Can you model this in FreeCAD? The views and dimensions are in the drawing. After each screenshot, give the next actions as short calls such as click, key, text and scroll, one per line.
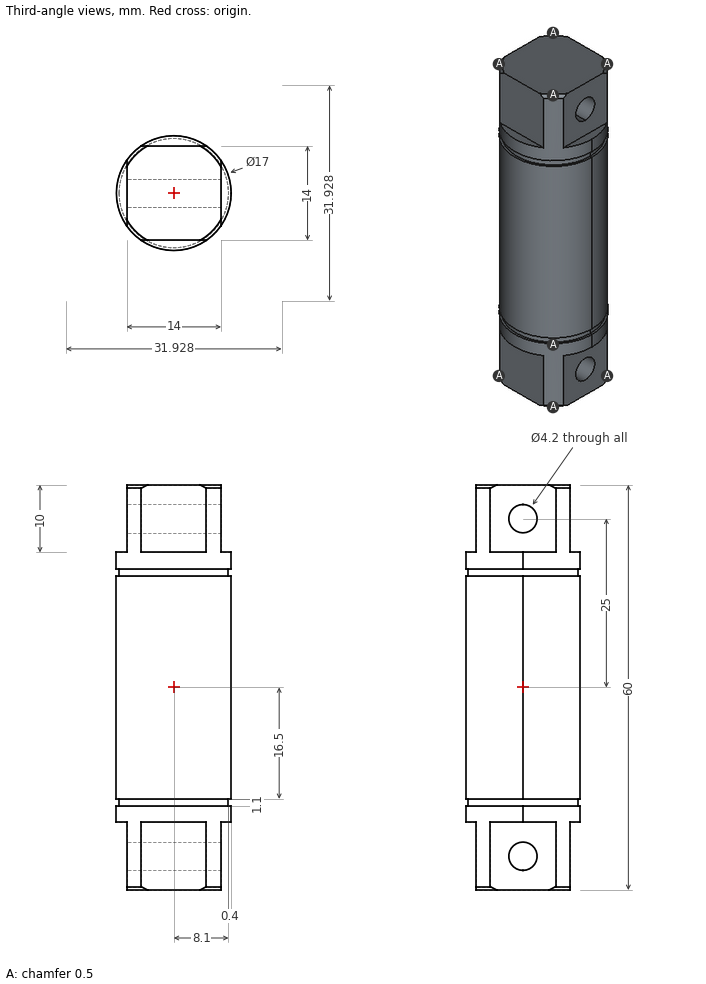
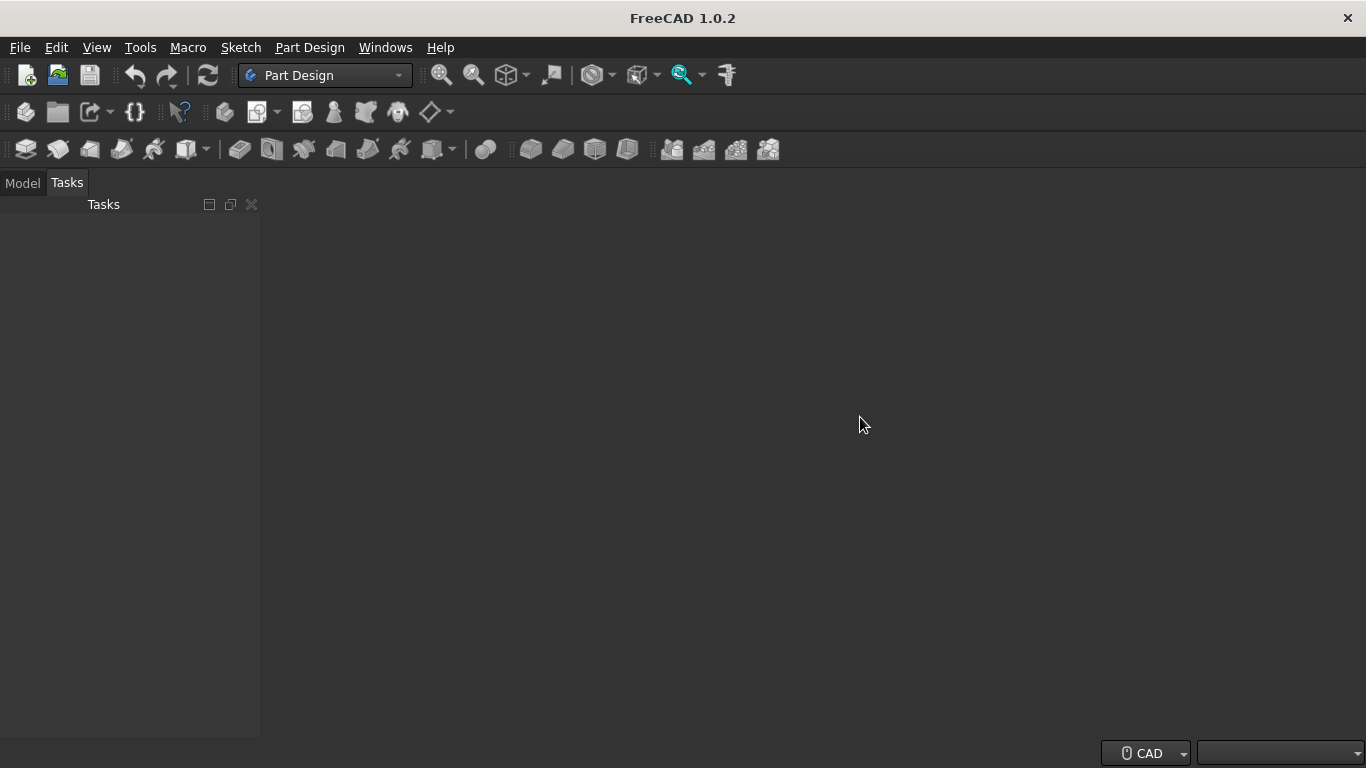
key(ctrl+n)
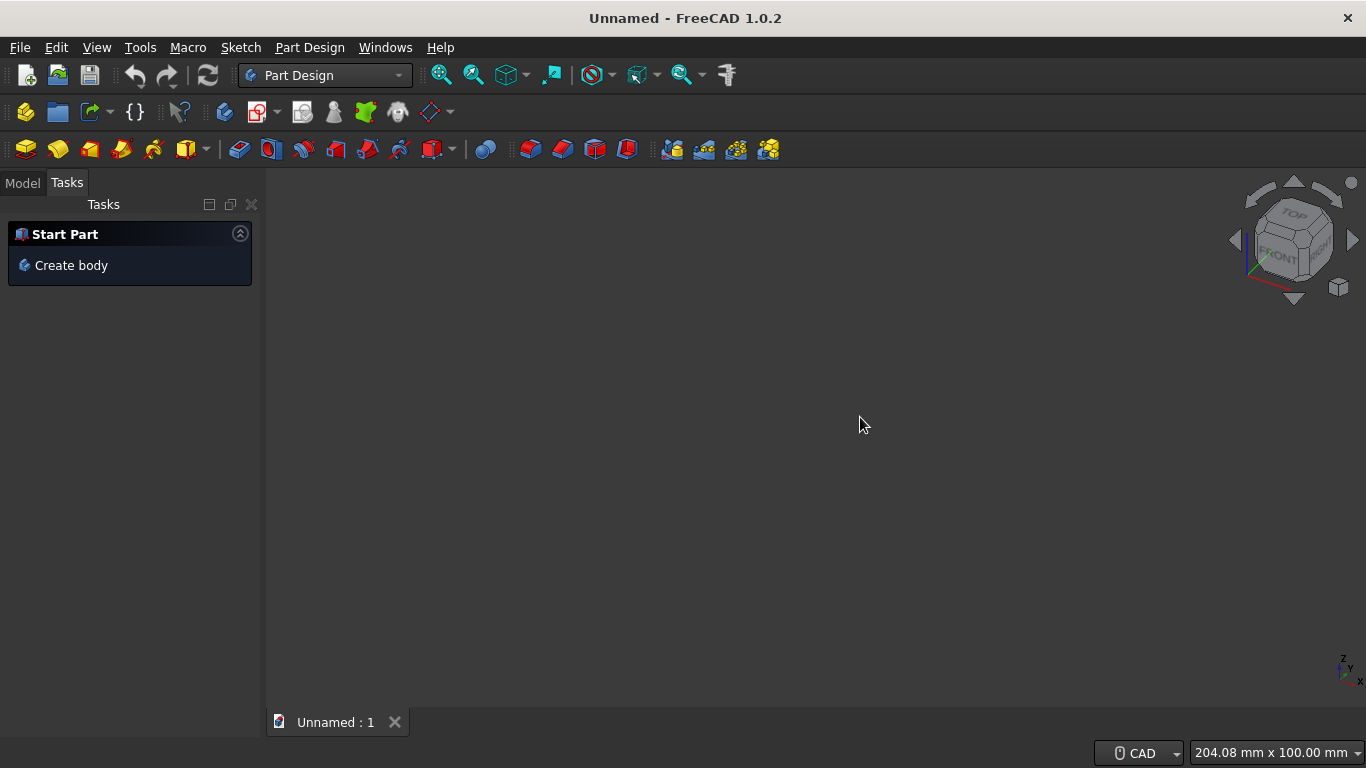
click(258, 112)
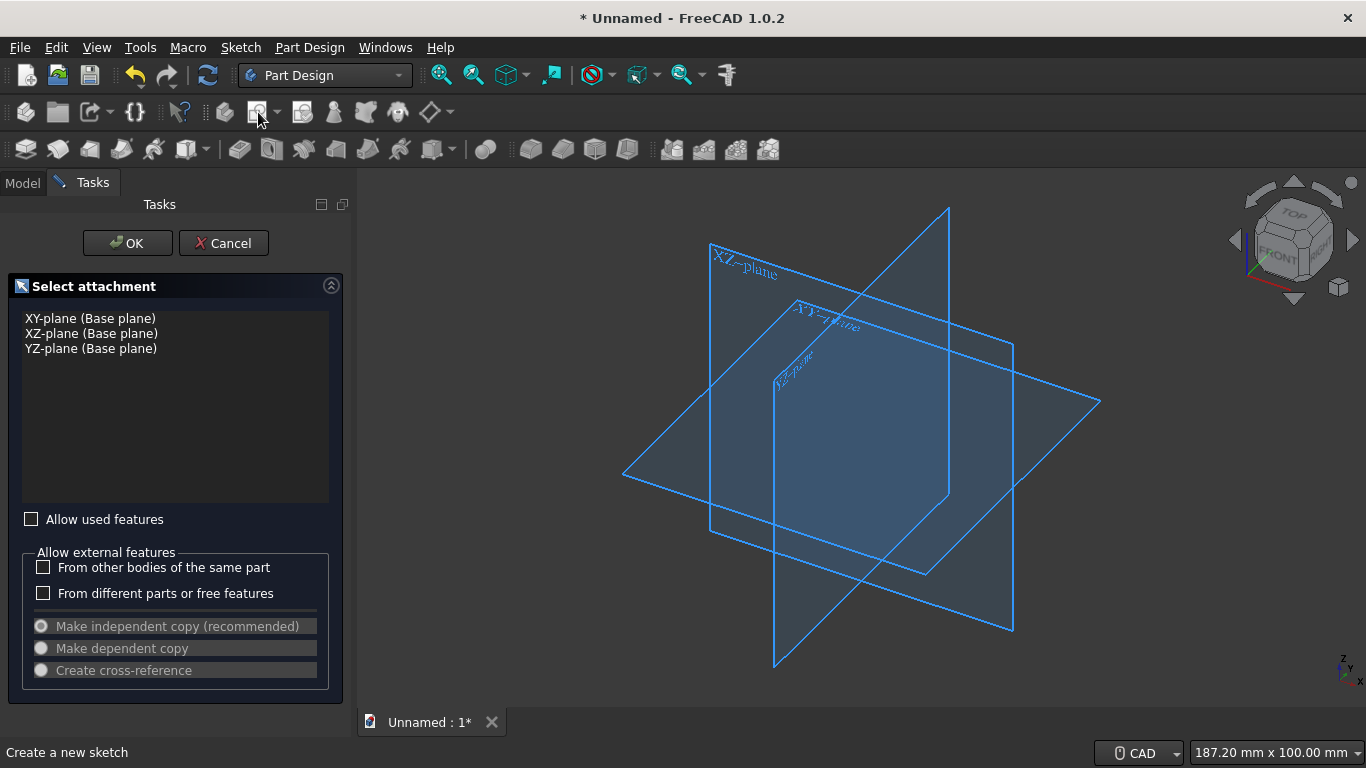
click(82, 318)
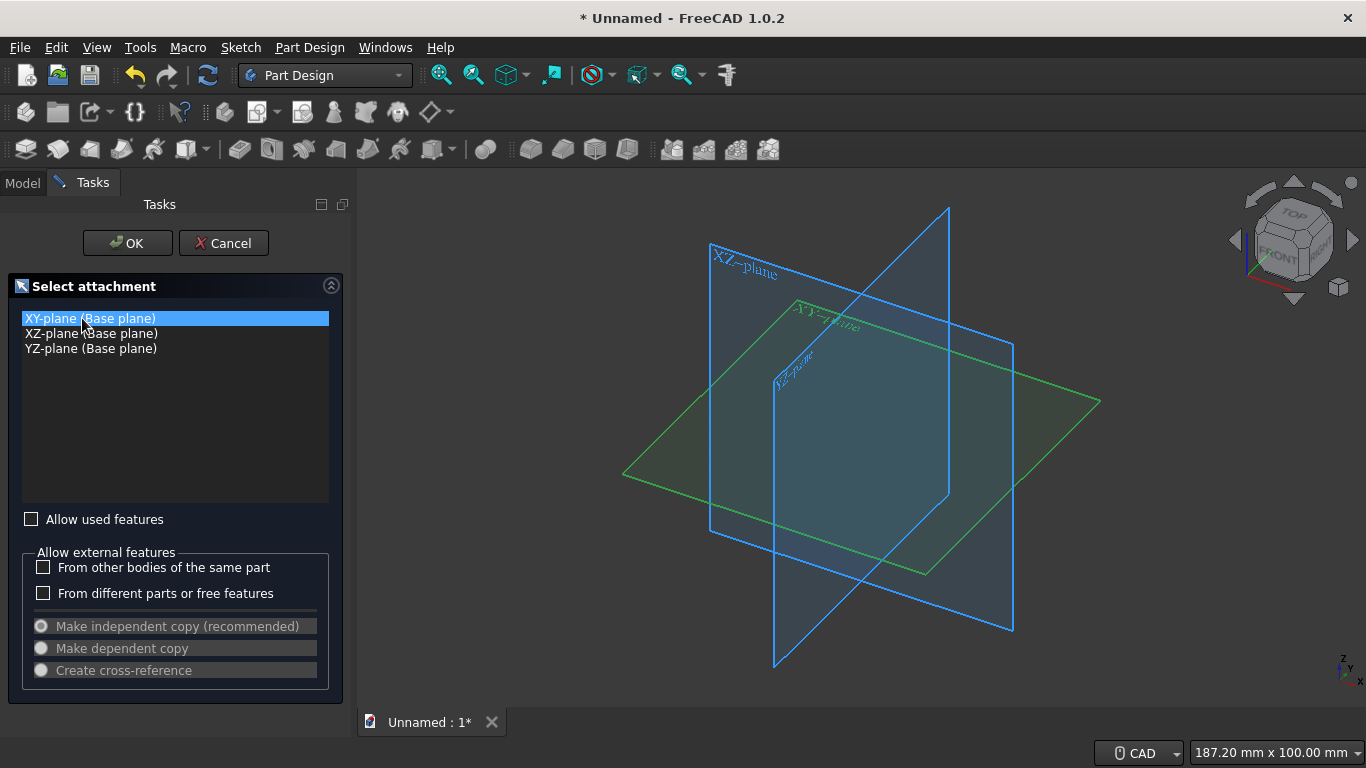
click(128, 243)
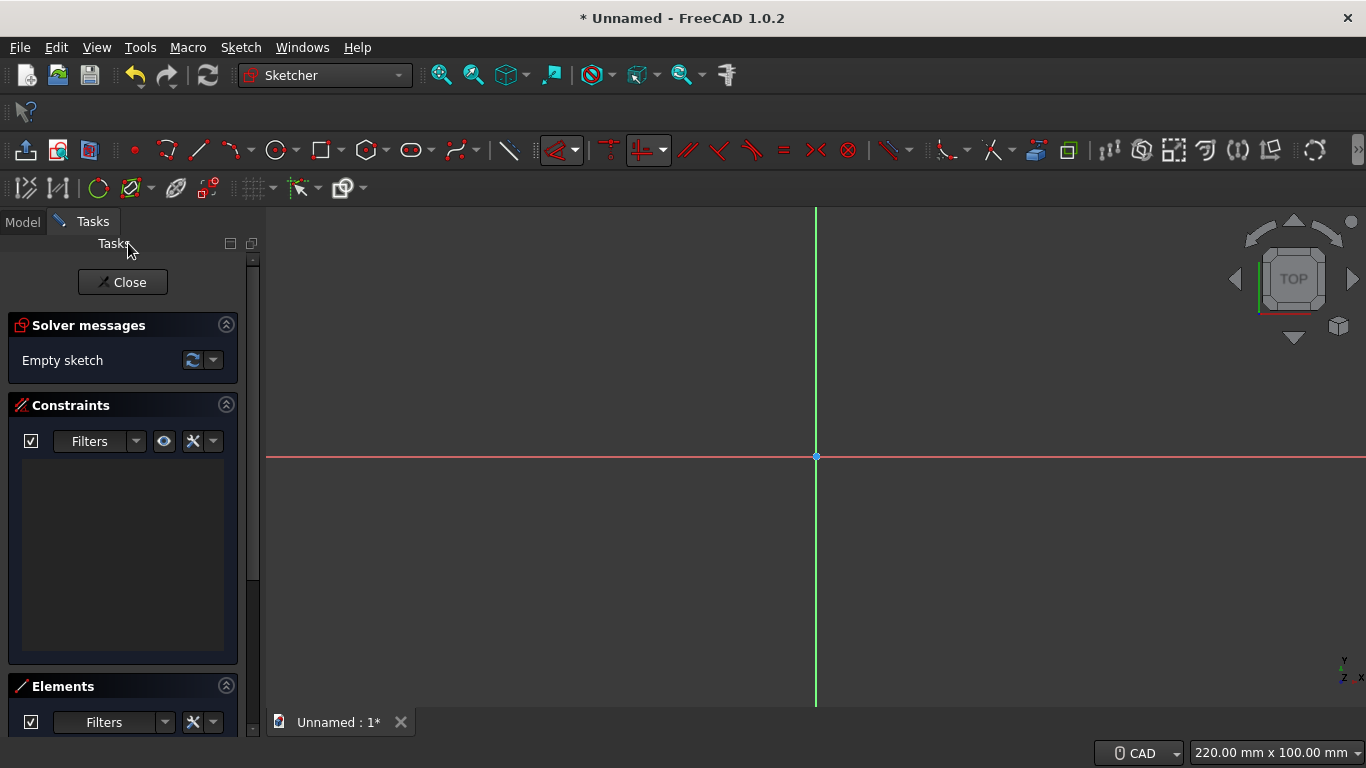
scroll(838, 457, up, 7)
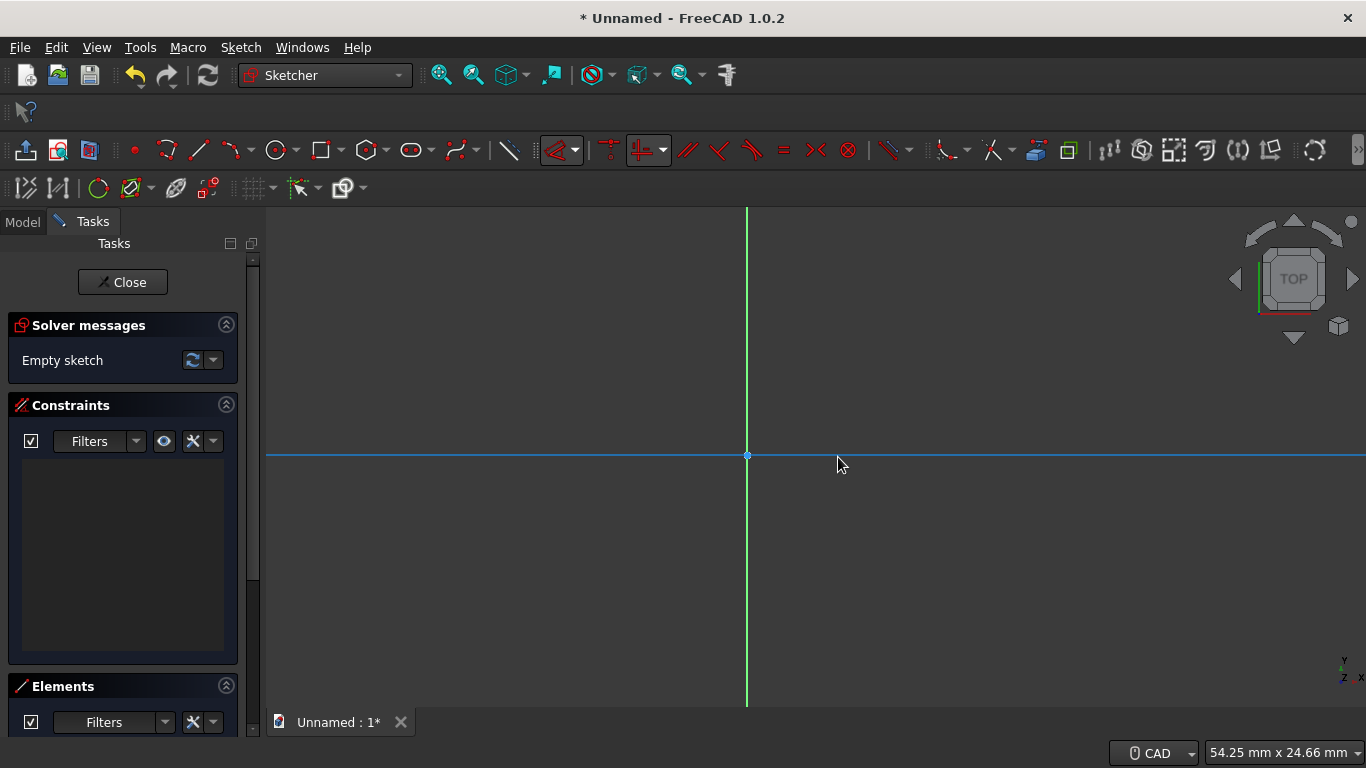
key(g)
key(c)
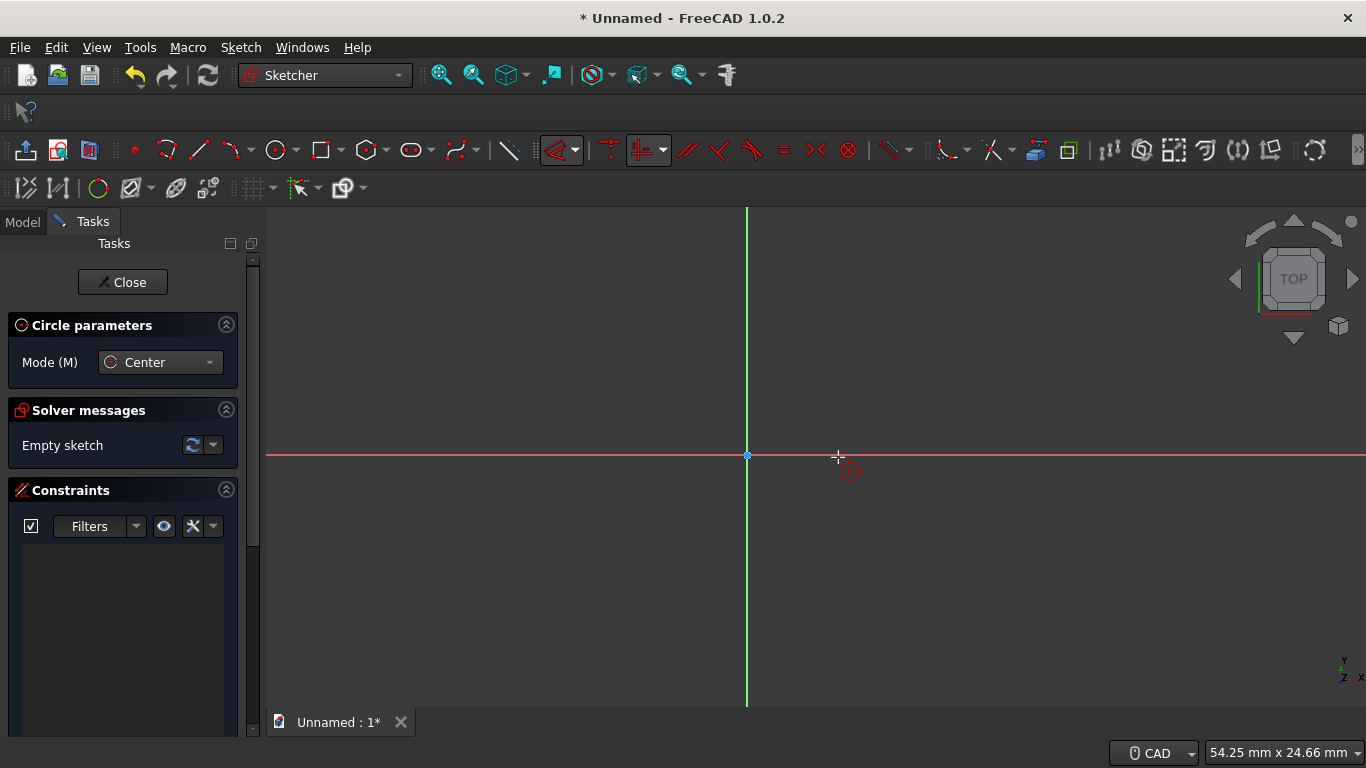
click(747, 455)
move(869, 334)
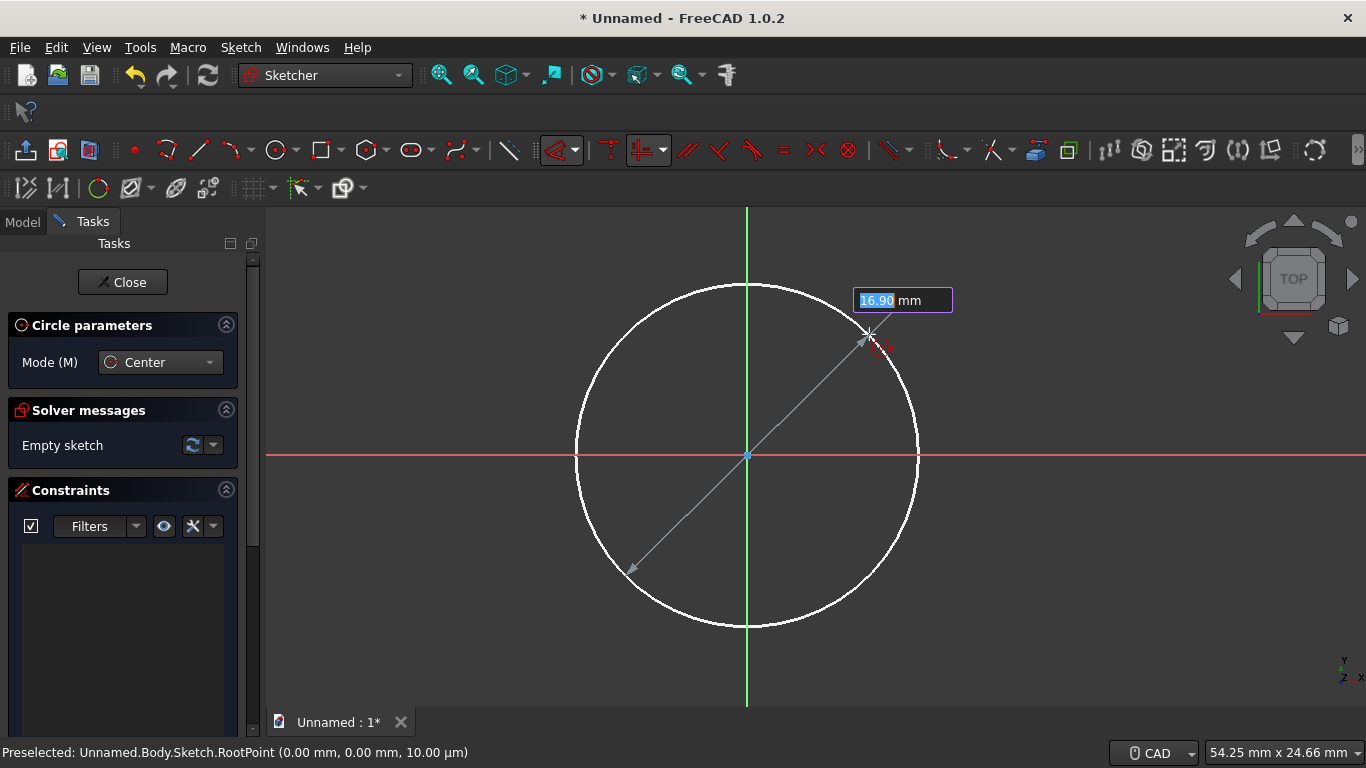
text(17)
key(Return)
key(Escape)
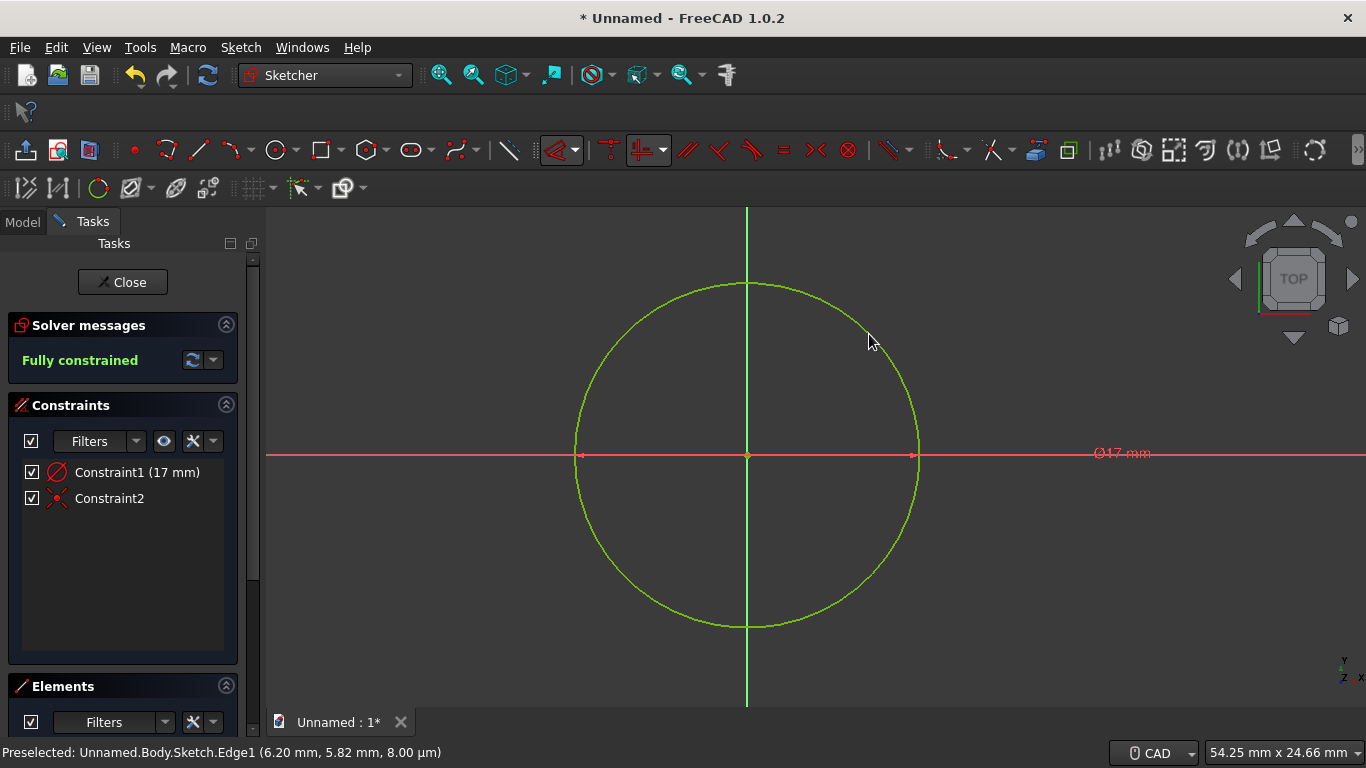
click(123, 282)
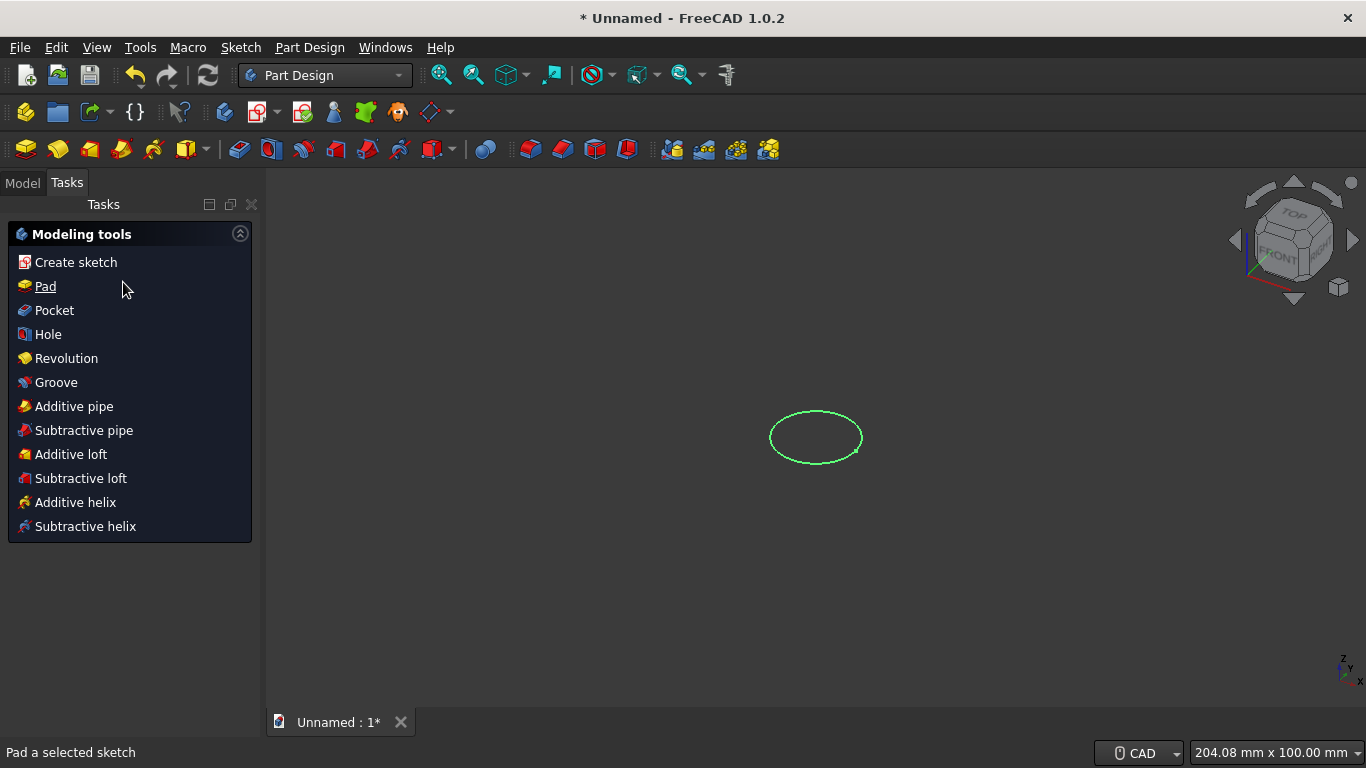
click(26, 150)